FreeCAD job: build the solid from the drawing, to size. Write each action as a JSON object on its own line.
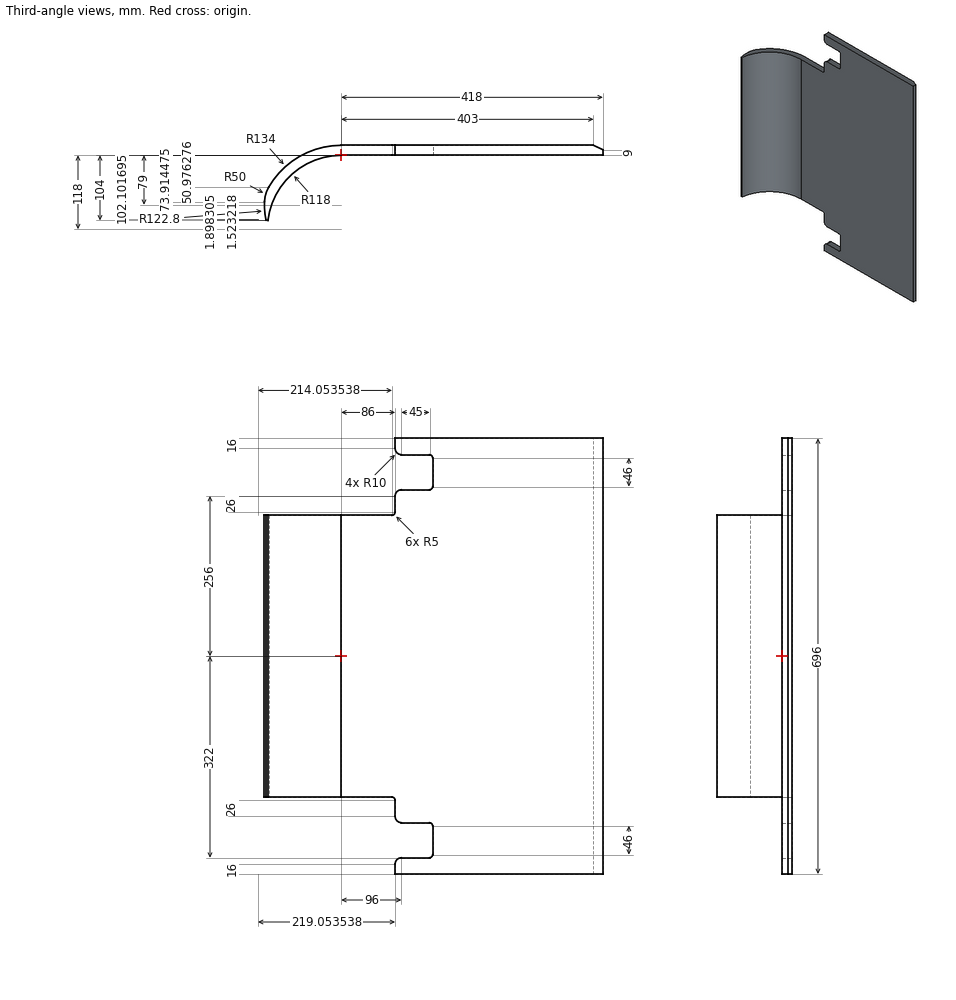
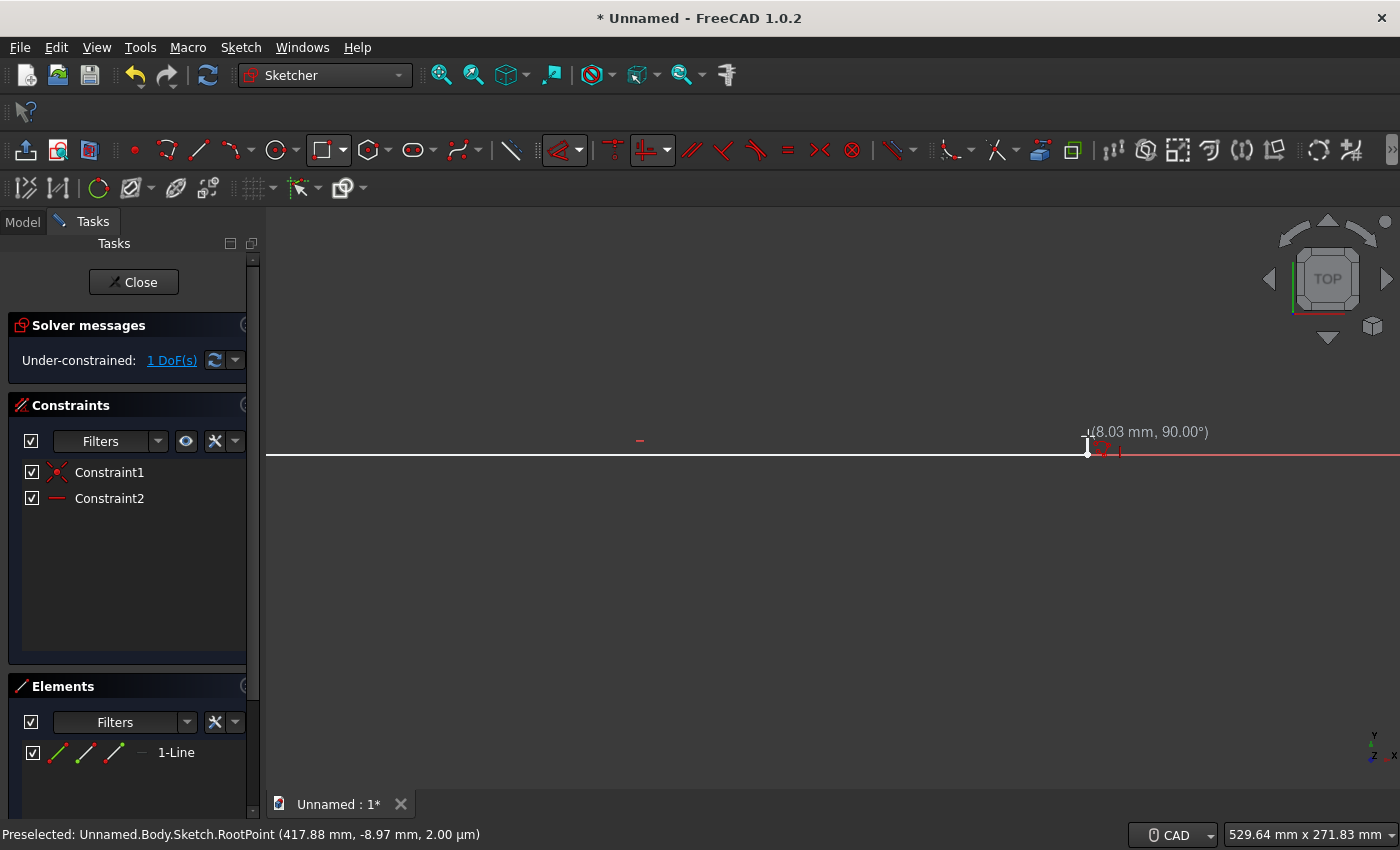
{"action": "left_click", "coordinate": [1087, 435]}
{"action": "left_click", "coordinate": [1056, 420]}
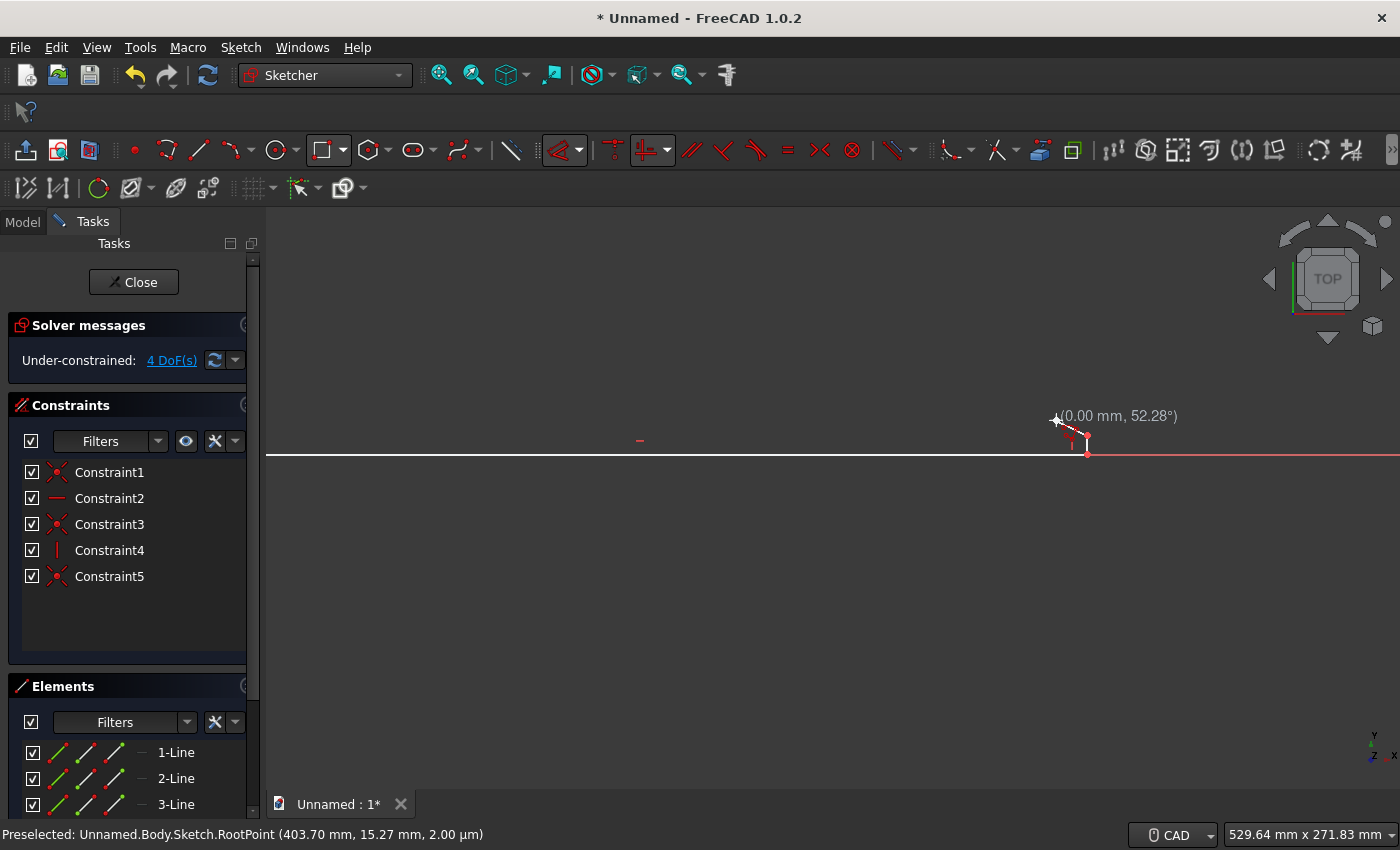
{"action": "scroll", "coordinate": [1089, 436], "scroll_direction": "down", "scroll_amount": 3}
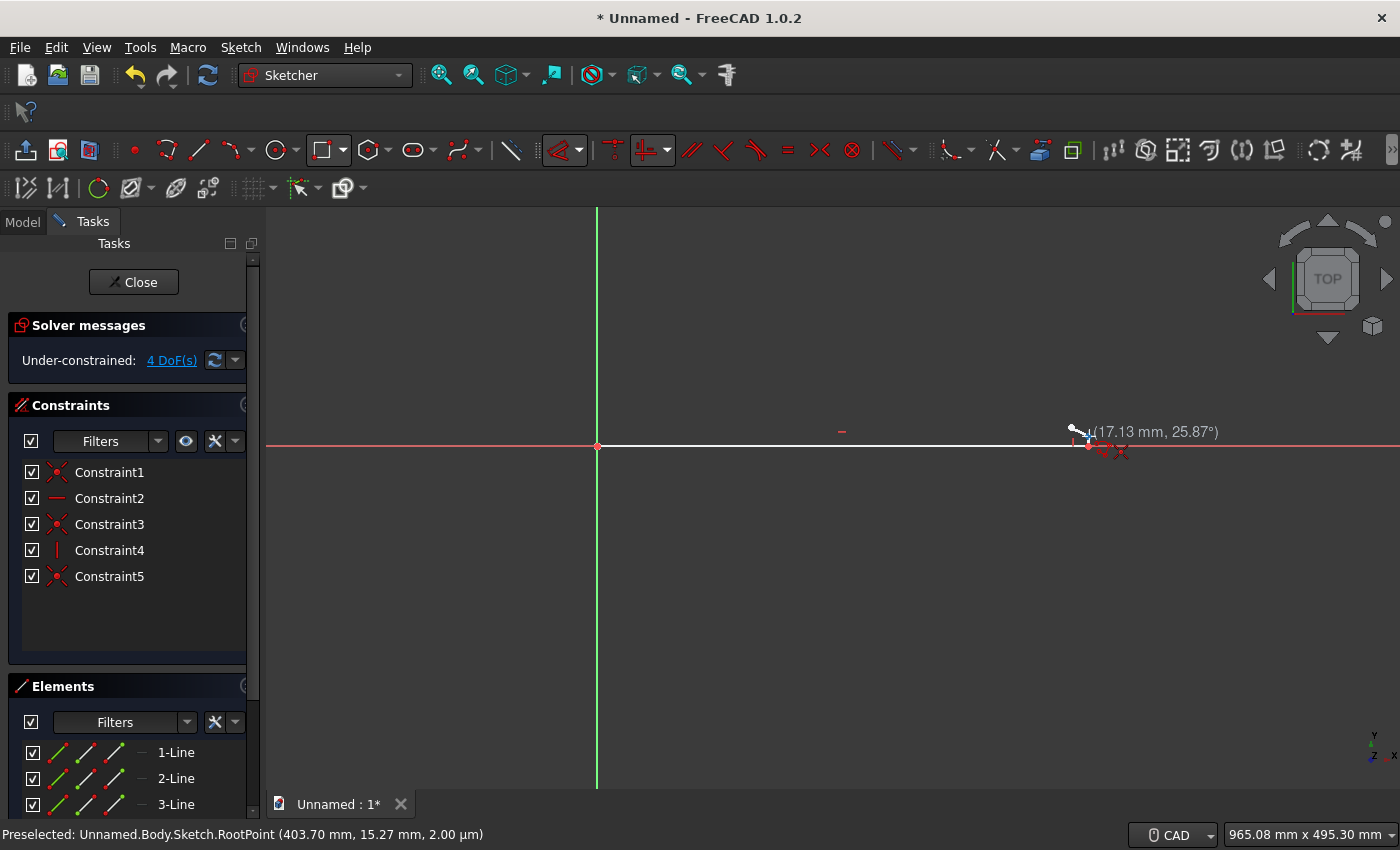
{"action": "left_click", "coordinate": [597, 427]}
{"action": "right_click", "coordinate": [597, 427]}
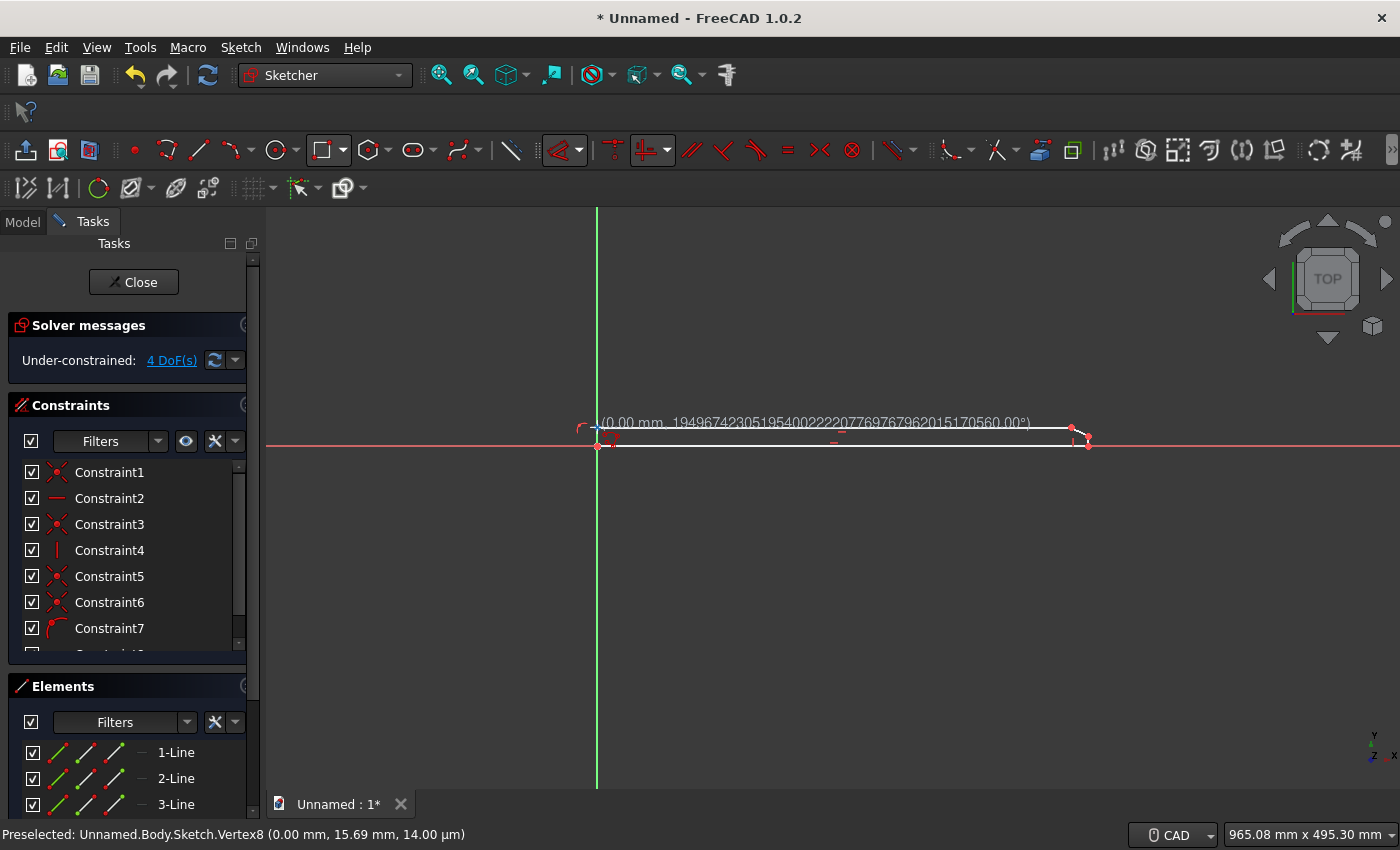
{"action": "left_click", "coordinate": [200, 150]}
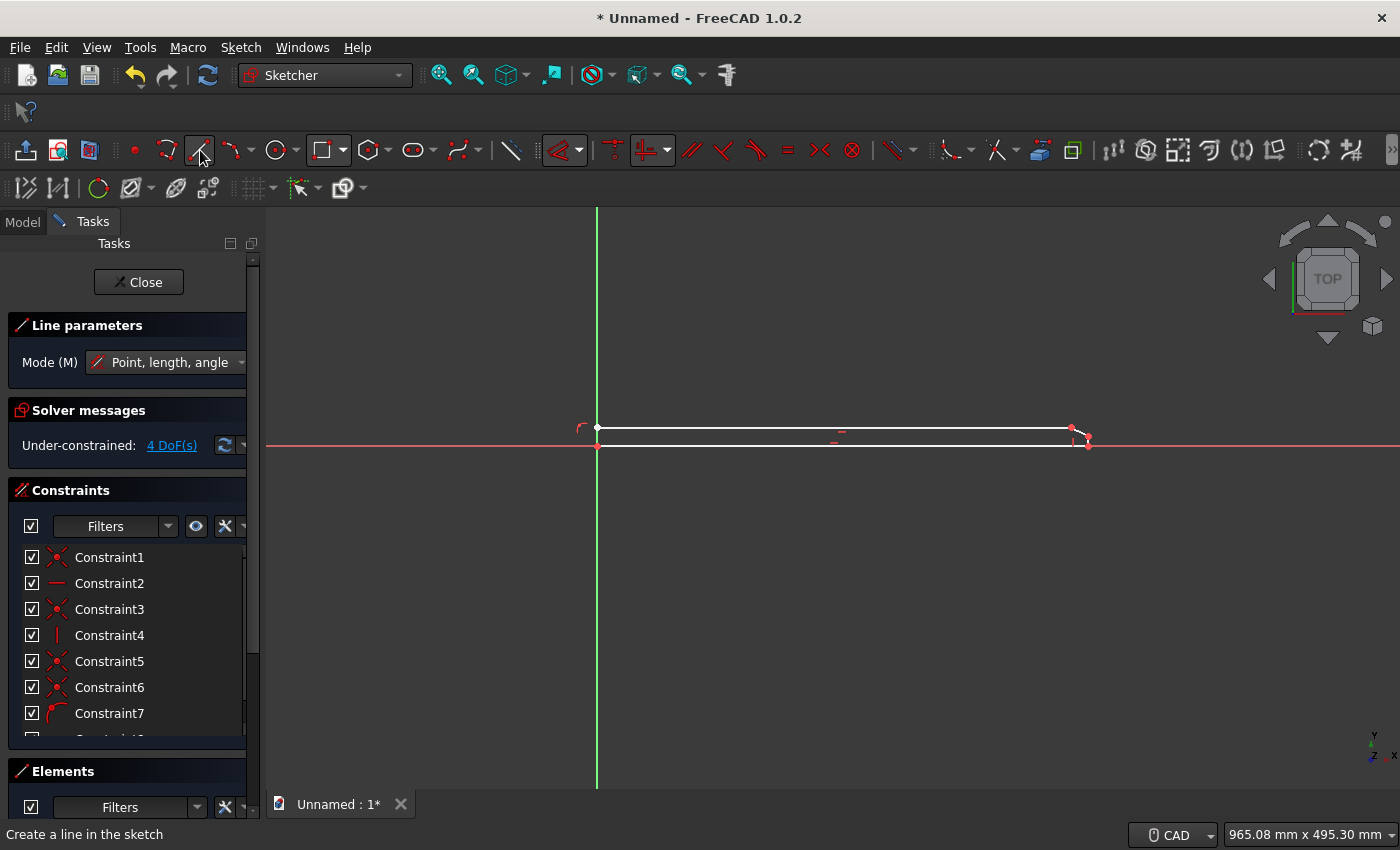
{"action": "left_click", "coordinate": [441, 566]}
{"action": "left_click", "coordinate": [460, 568]}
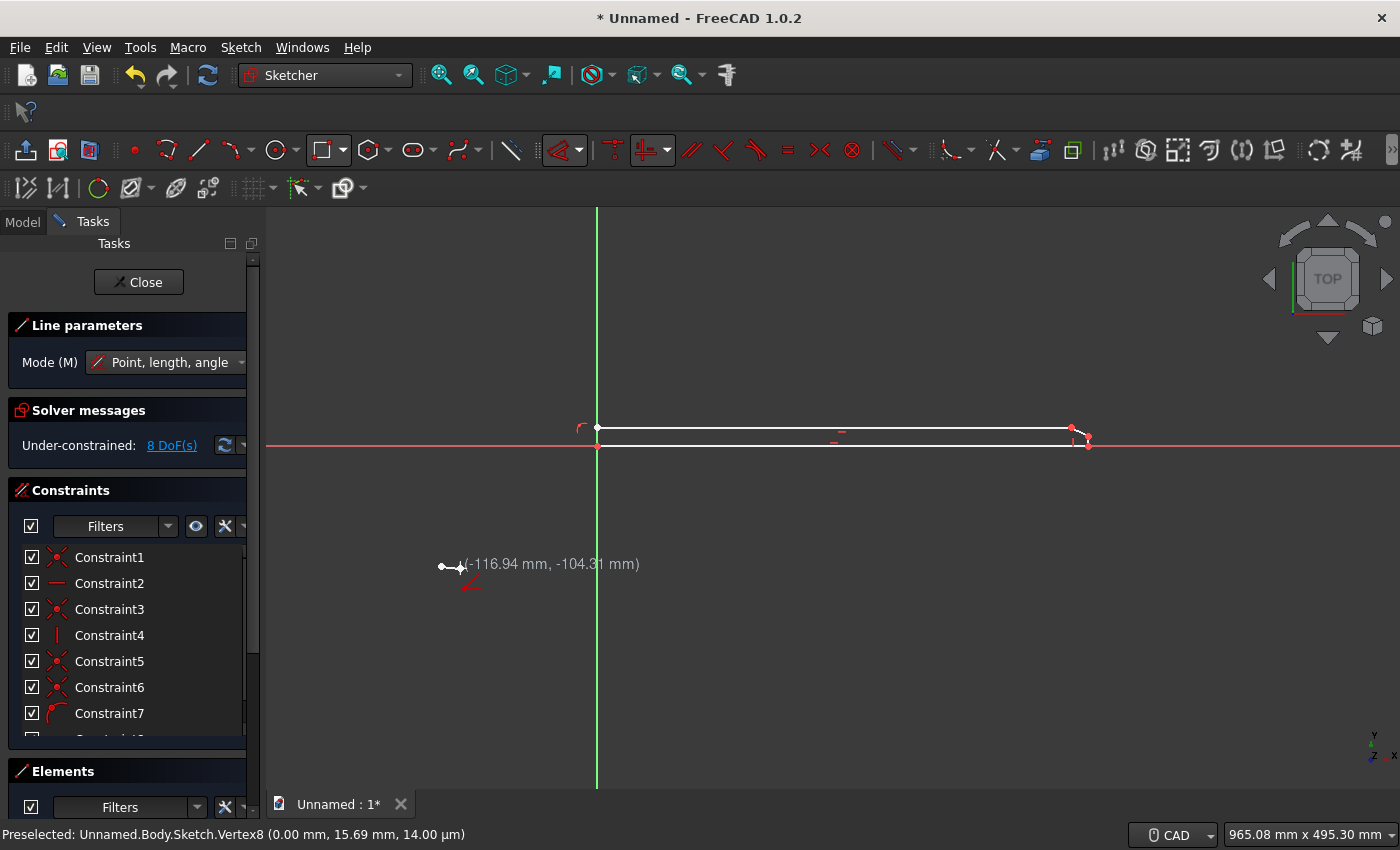
{"action": "left_click", "coordinate": [232, 150]}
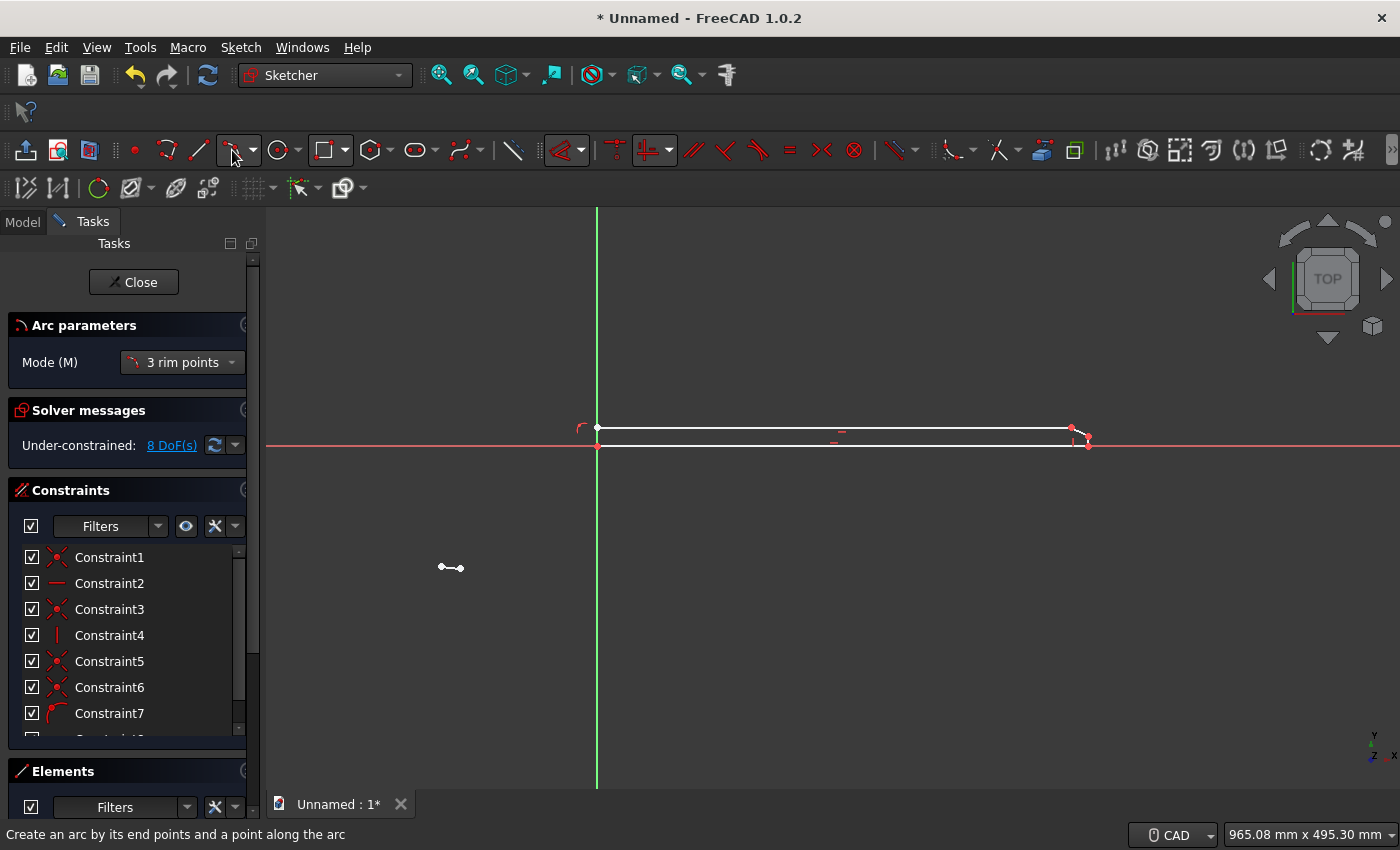
{"action": "left_click", "coordinate": [597, 428]}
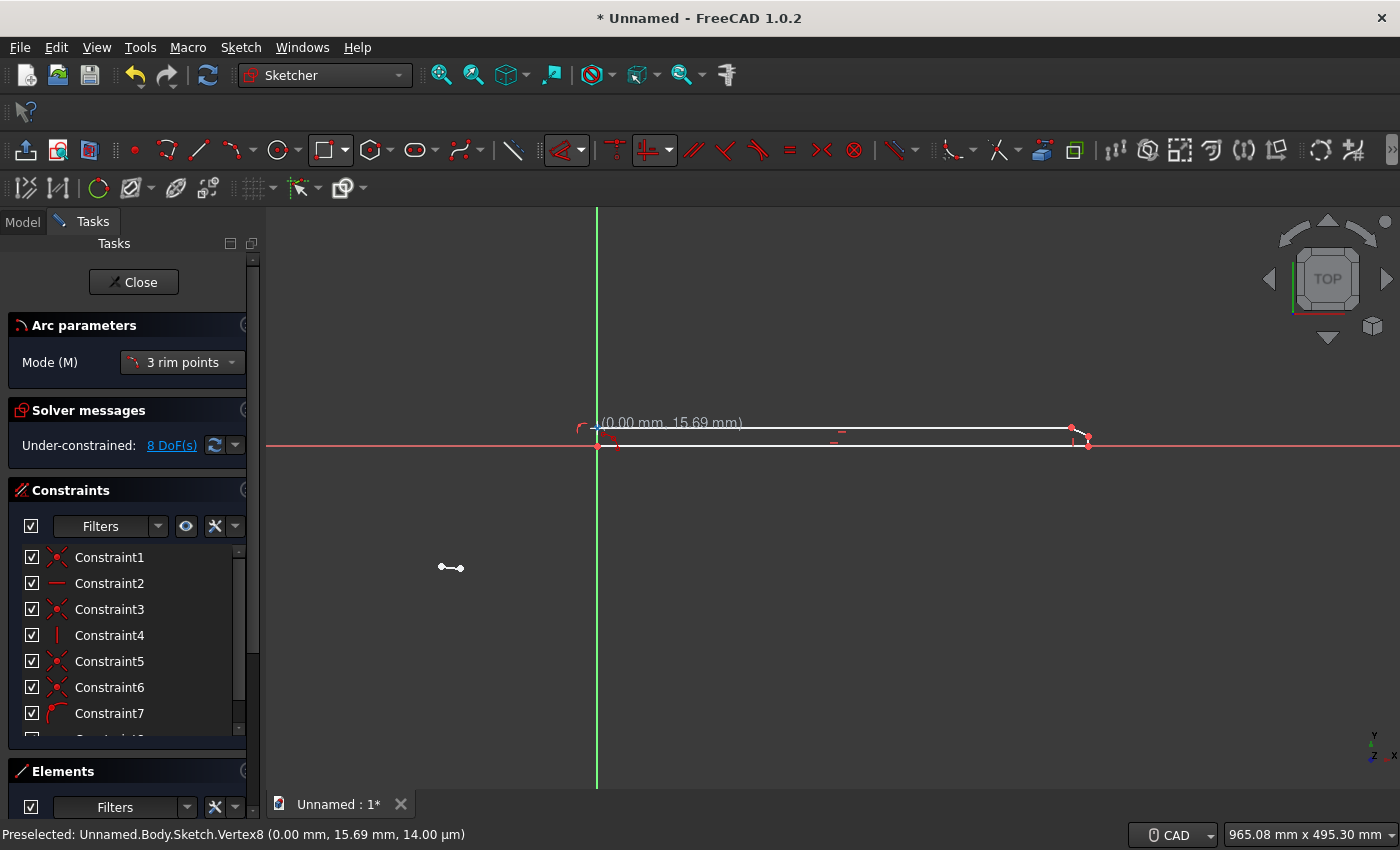
{"action": "scroll", "coordinate": [441, 566], "scroll_direction": "up", "scroll_amount": 3}